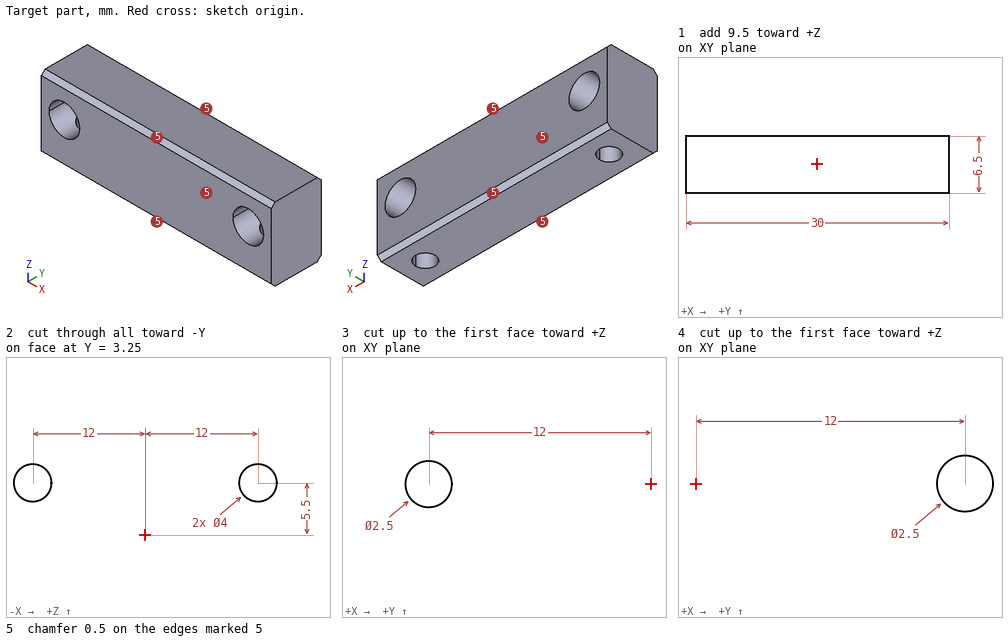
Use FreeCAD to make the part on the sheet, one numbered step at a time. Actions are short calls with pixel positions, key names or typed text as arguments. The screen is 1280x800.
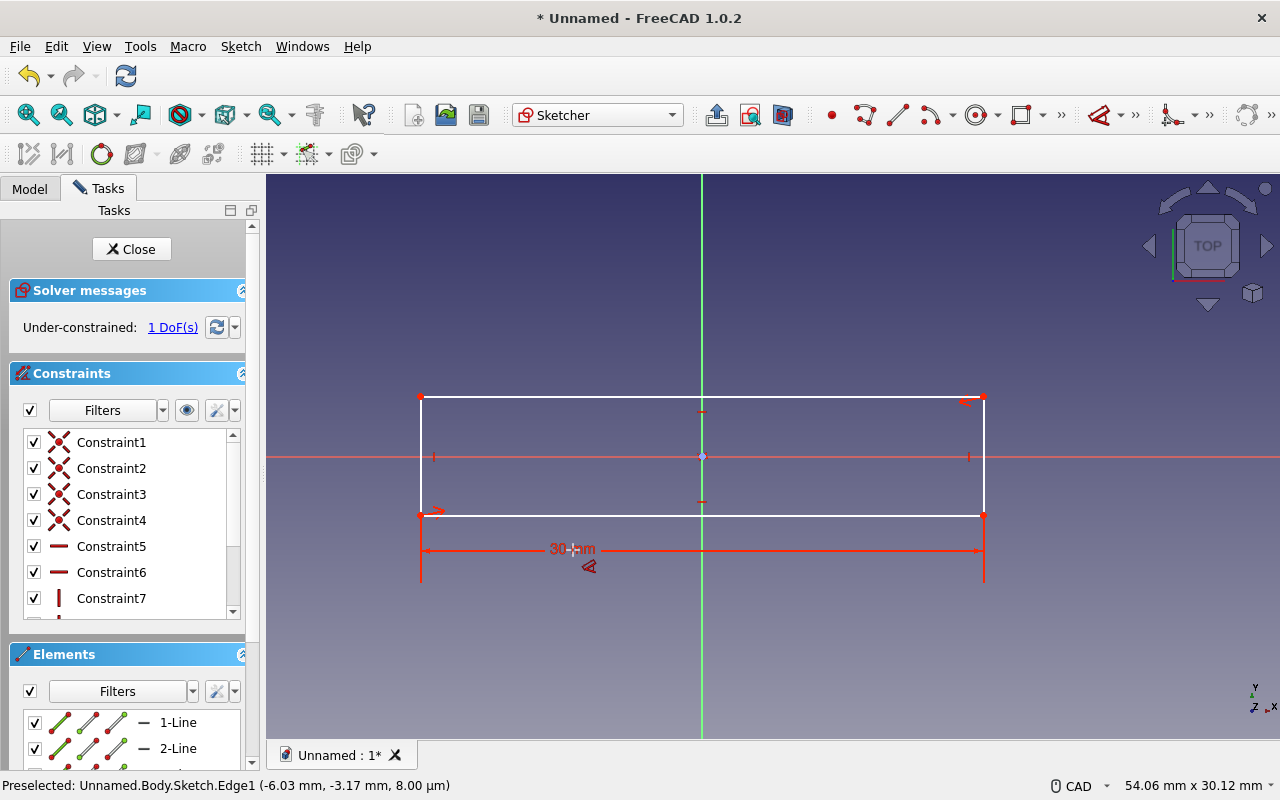
click(984, 480)
click(1018, 429)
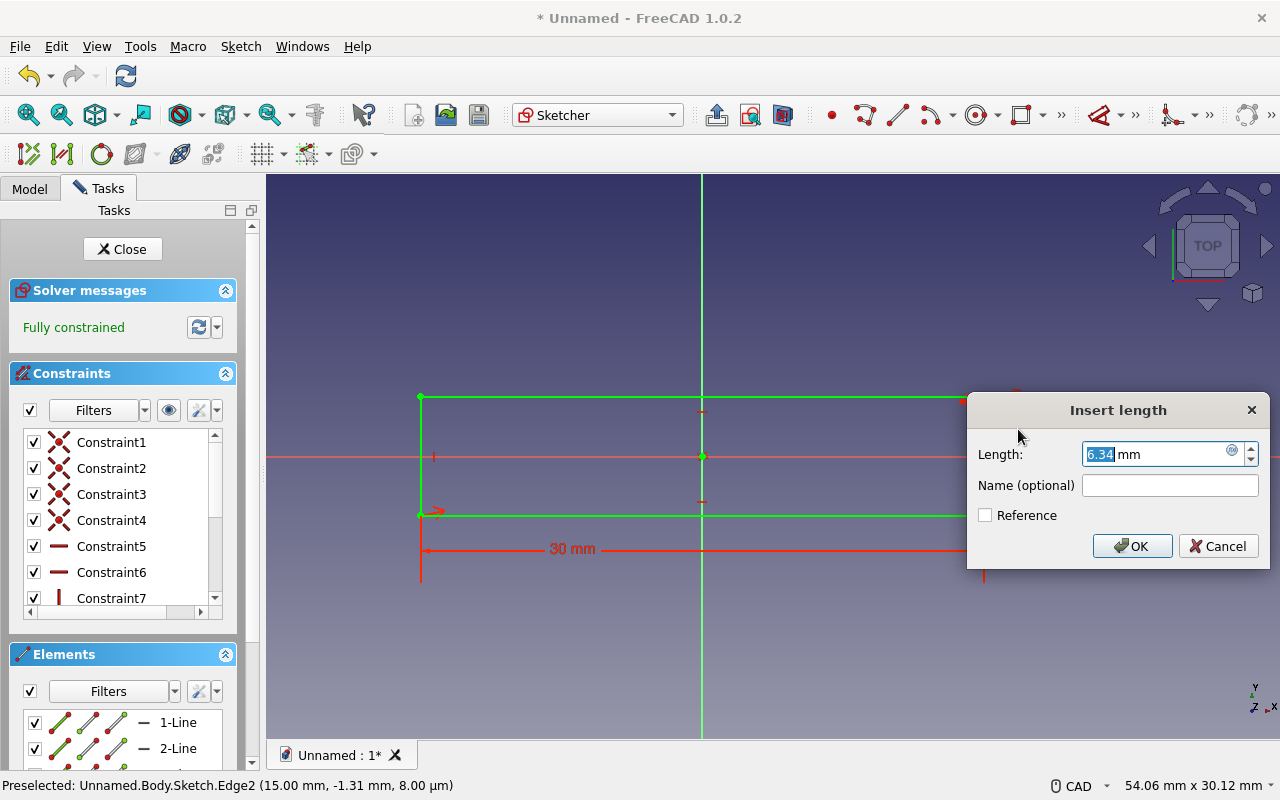
text(6.5)
key(Return)
key(Escape)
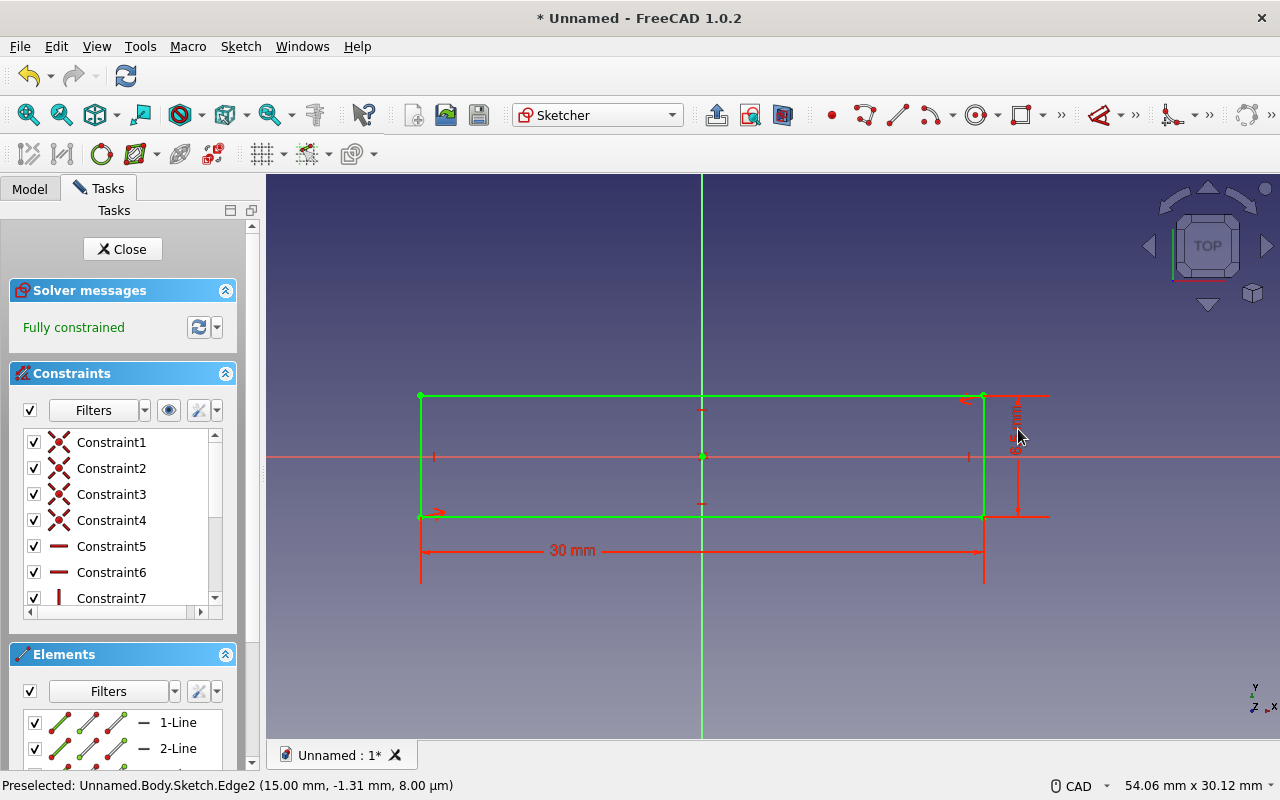
click(123, 249)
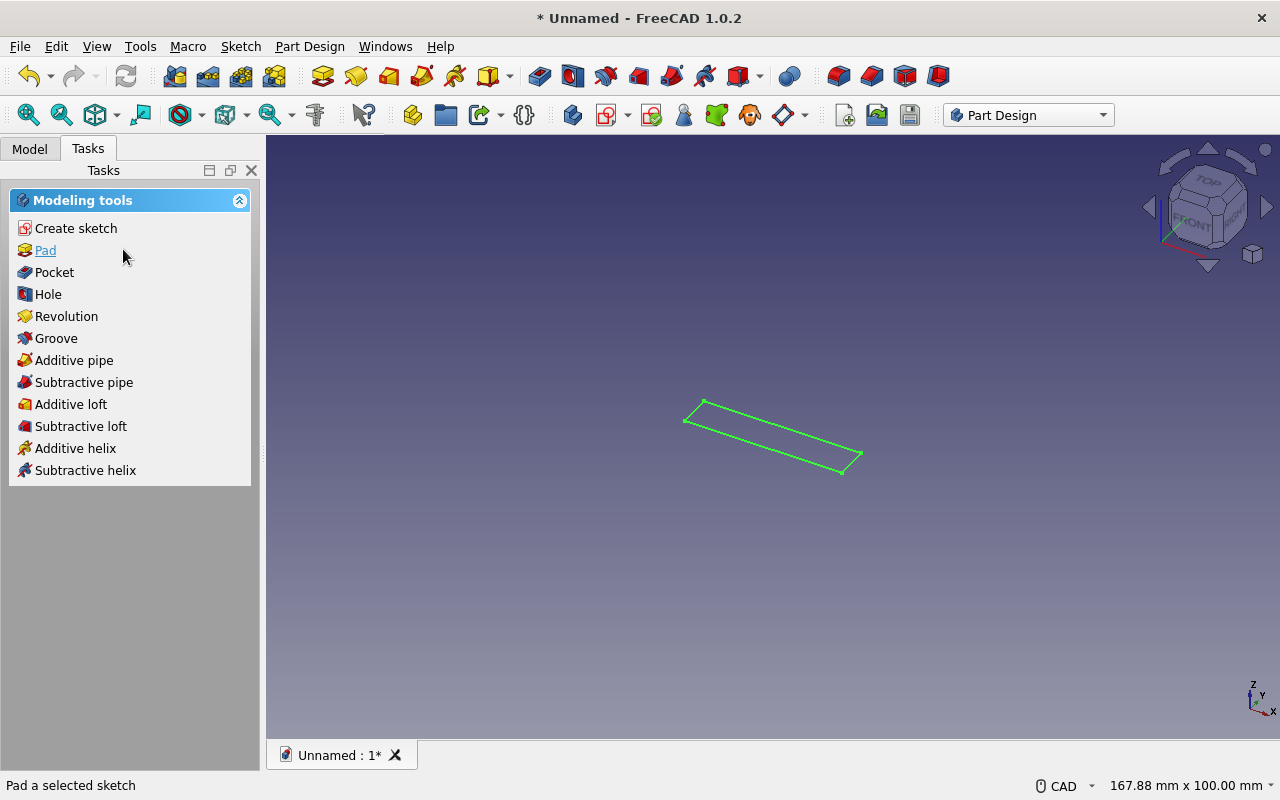
click(323, 76)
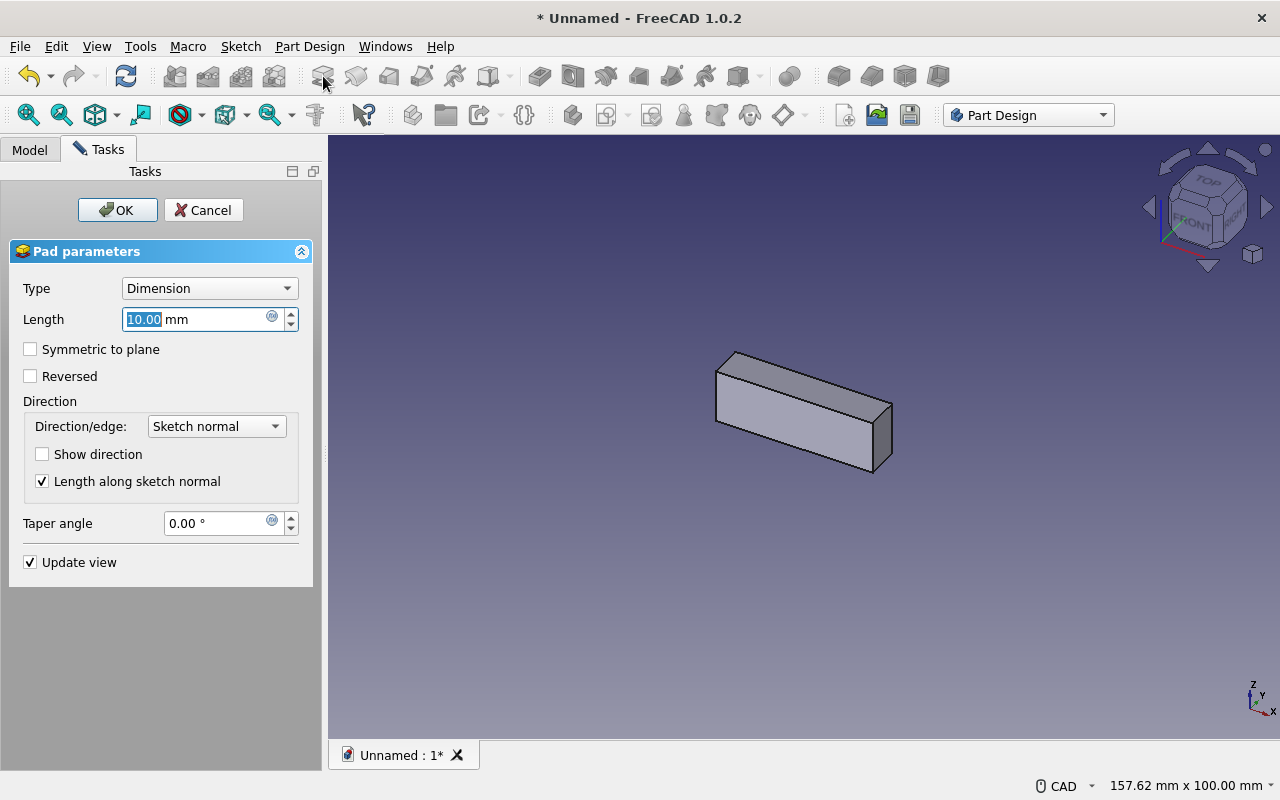
text(9.5)
key(Tab)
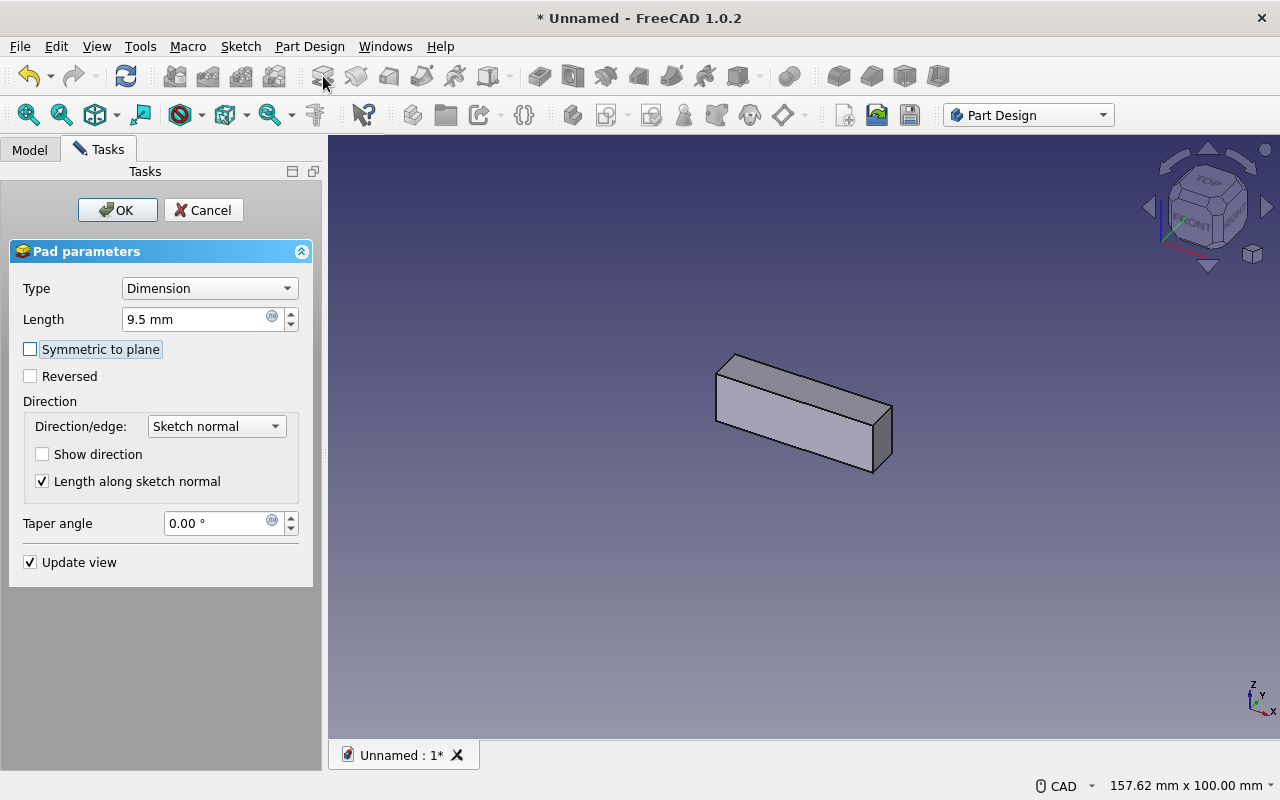
click(118, 210)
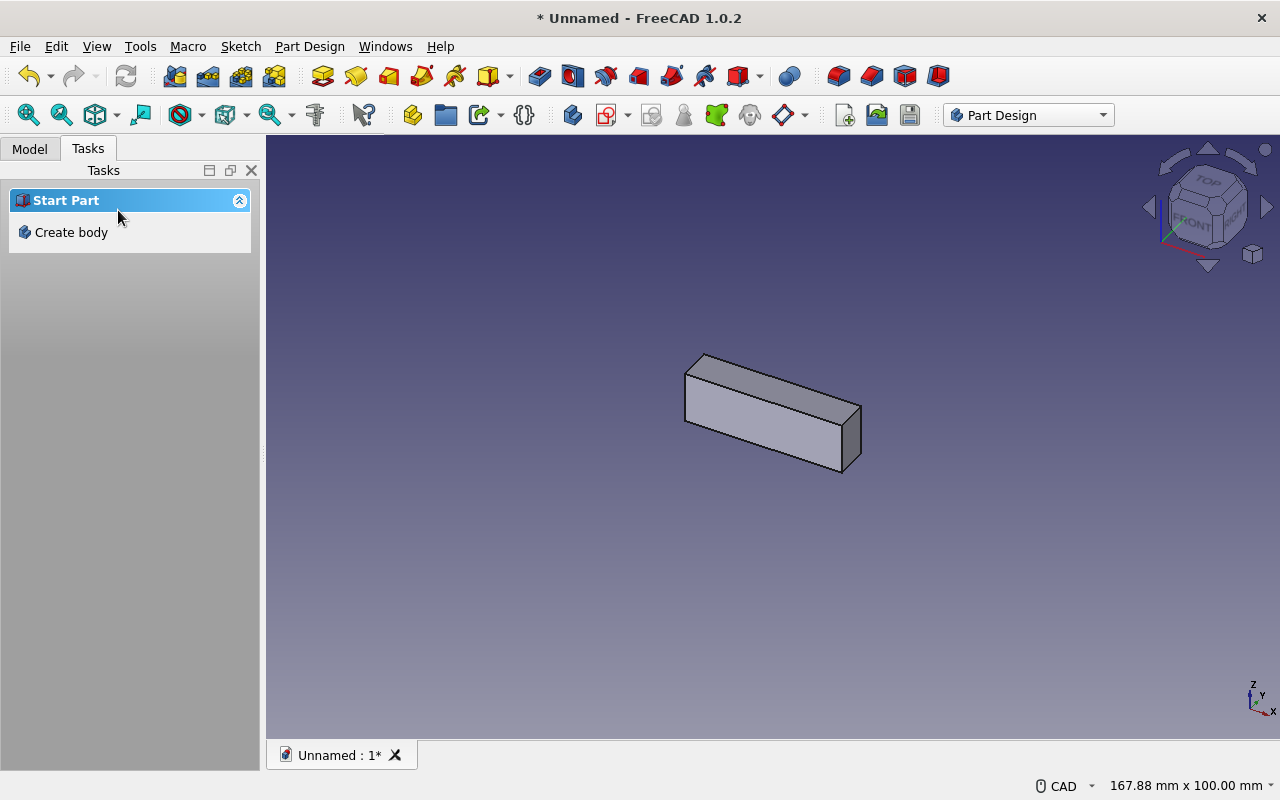
key(v)
key(f)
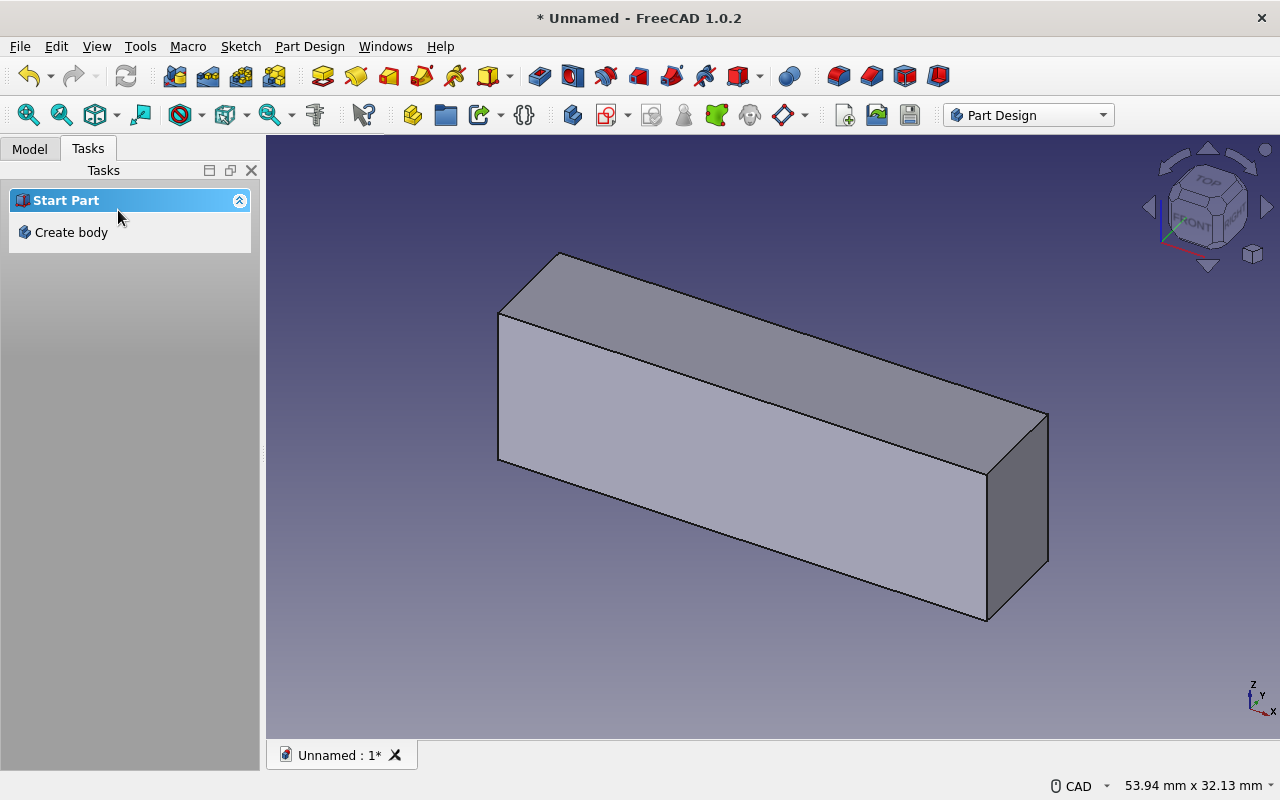
key(4)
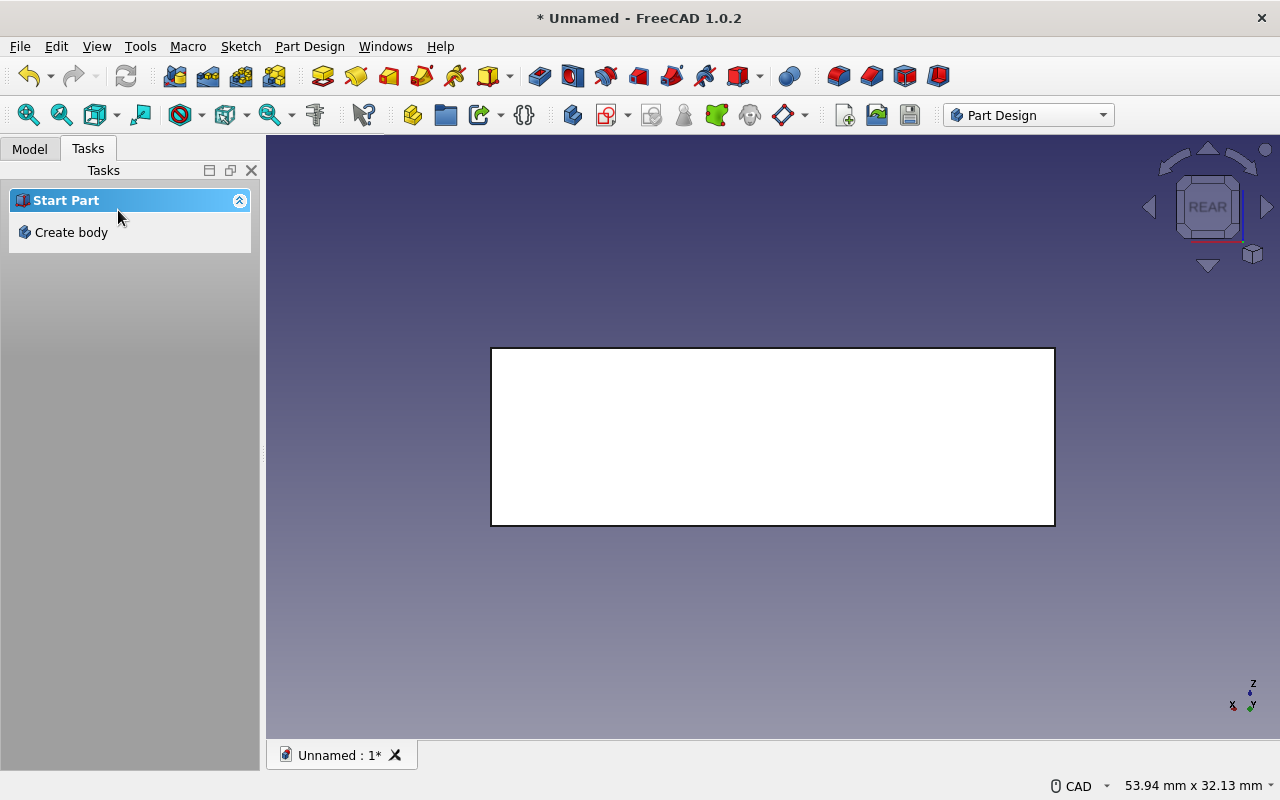
click(612, 436)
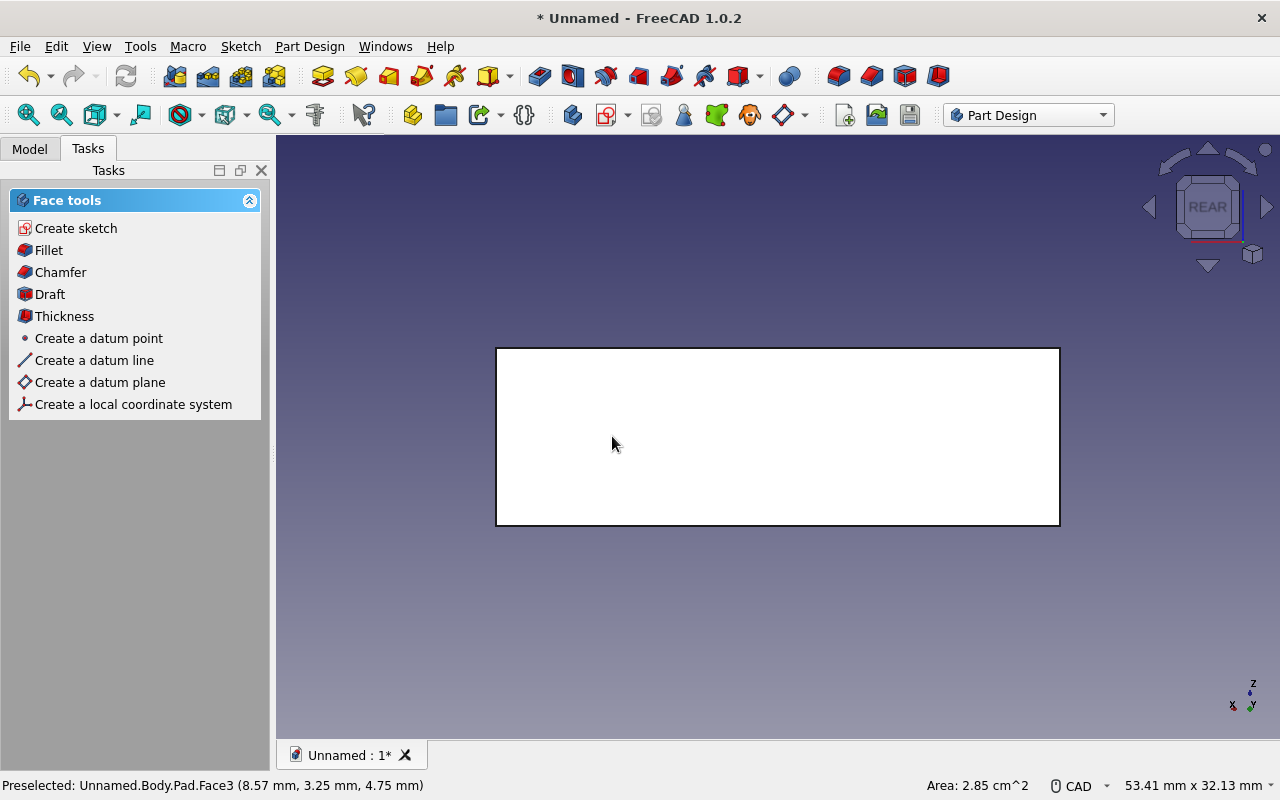
click(606, 116)